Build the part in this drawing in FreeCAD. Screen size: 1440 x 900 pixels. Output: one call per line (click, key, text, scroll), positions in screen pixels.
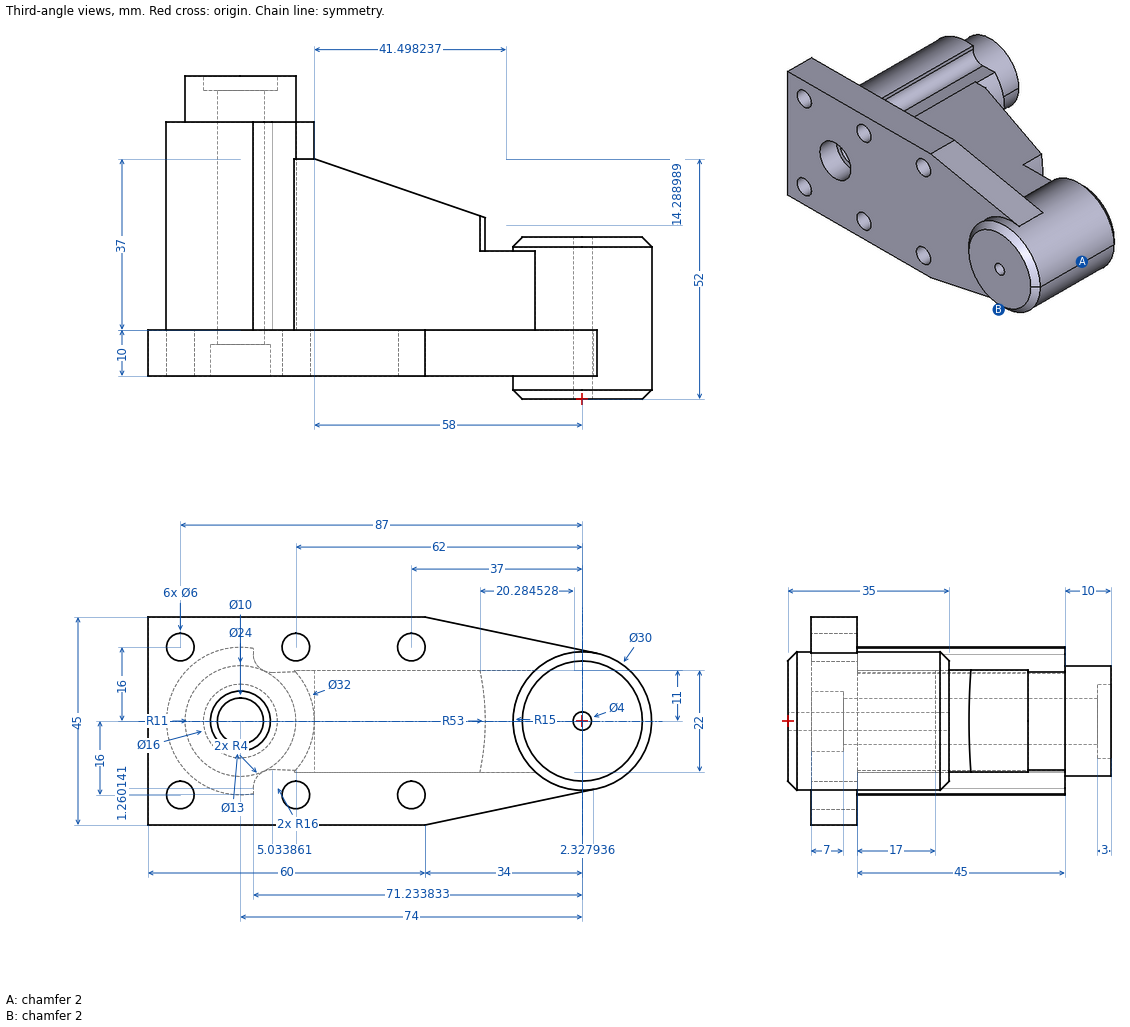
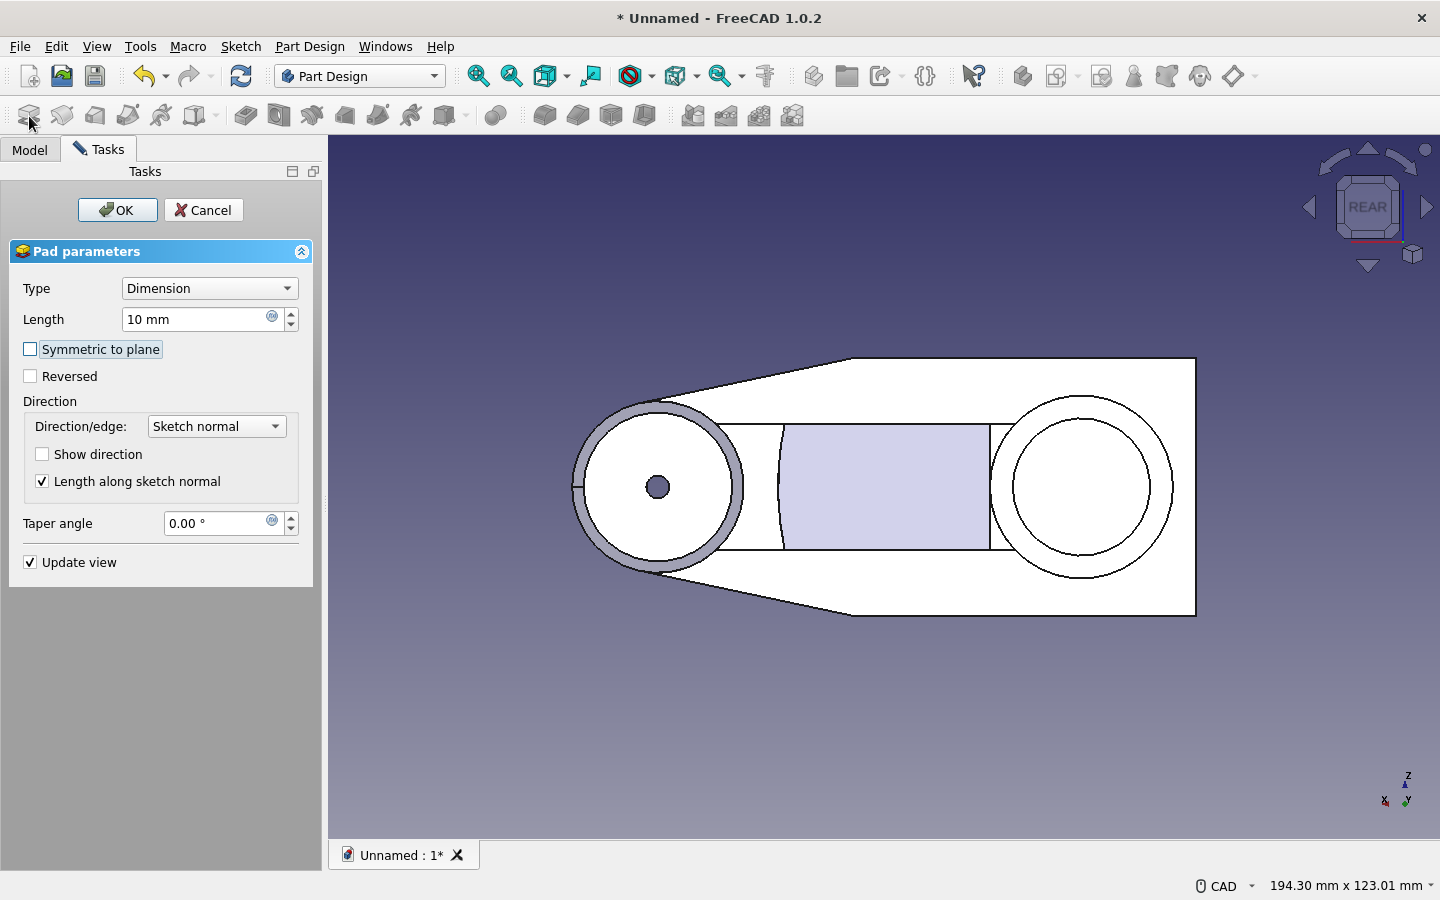
click(118, 210)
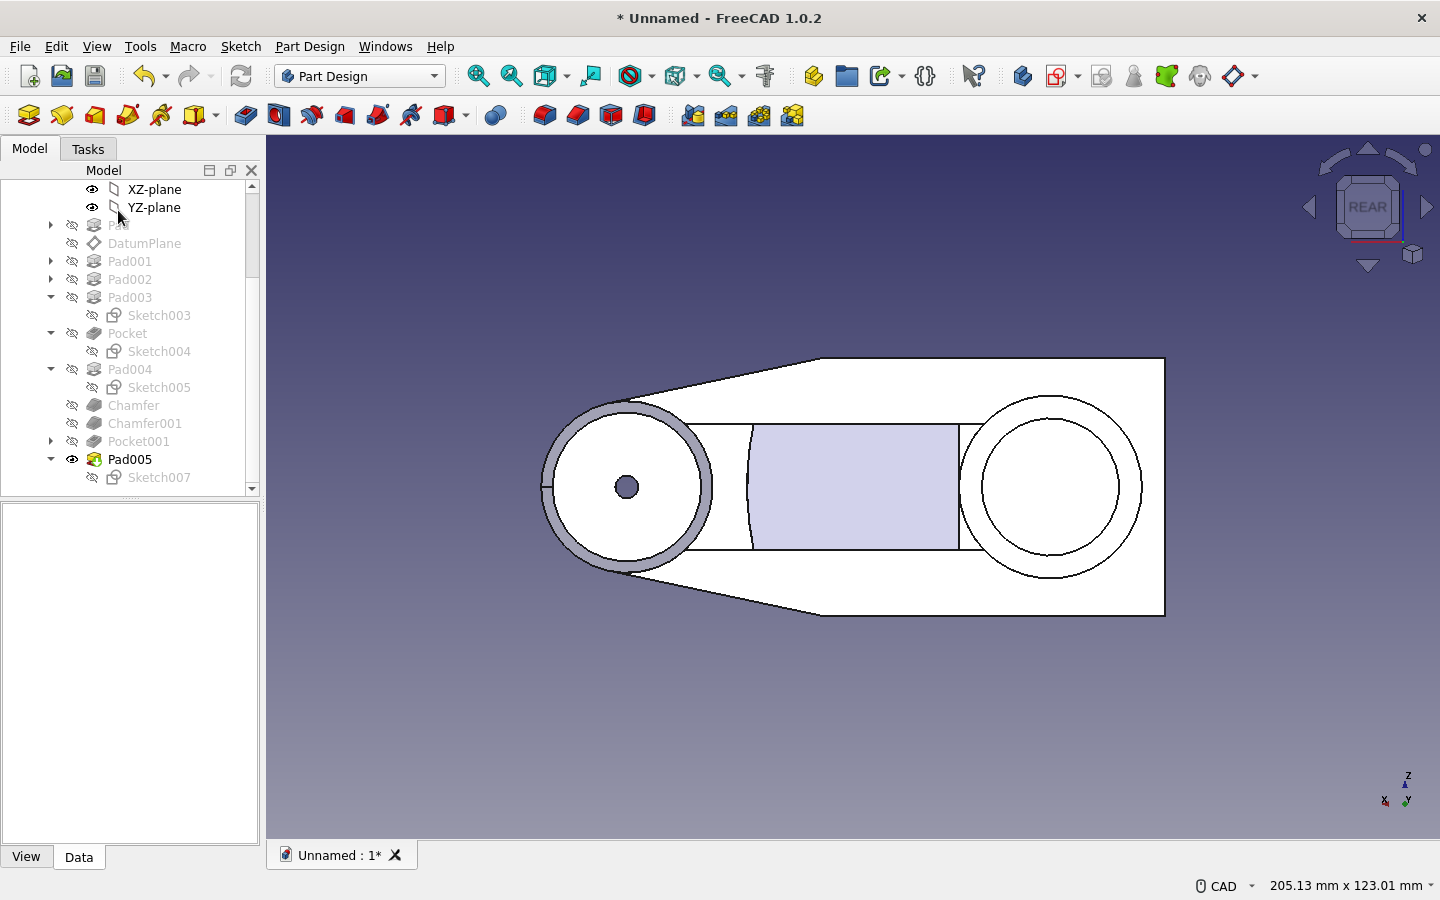
click(1050, 486)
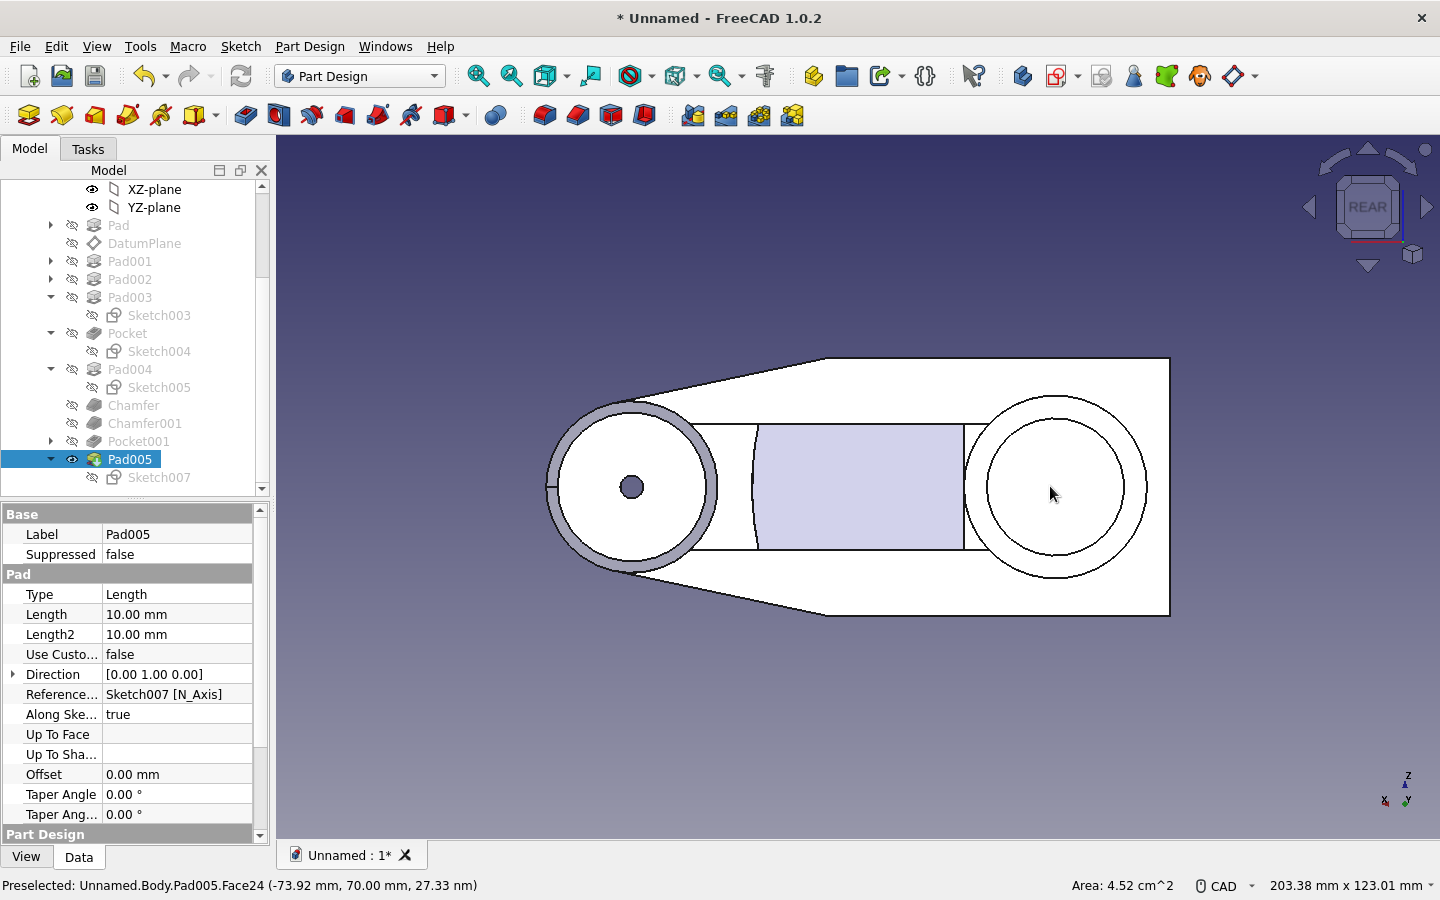
click(1056, 76)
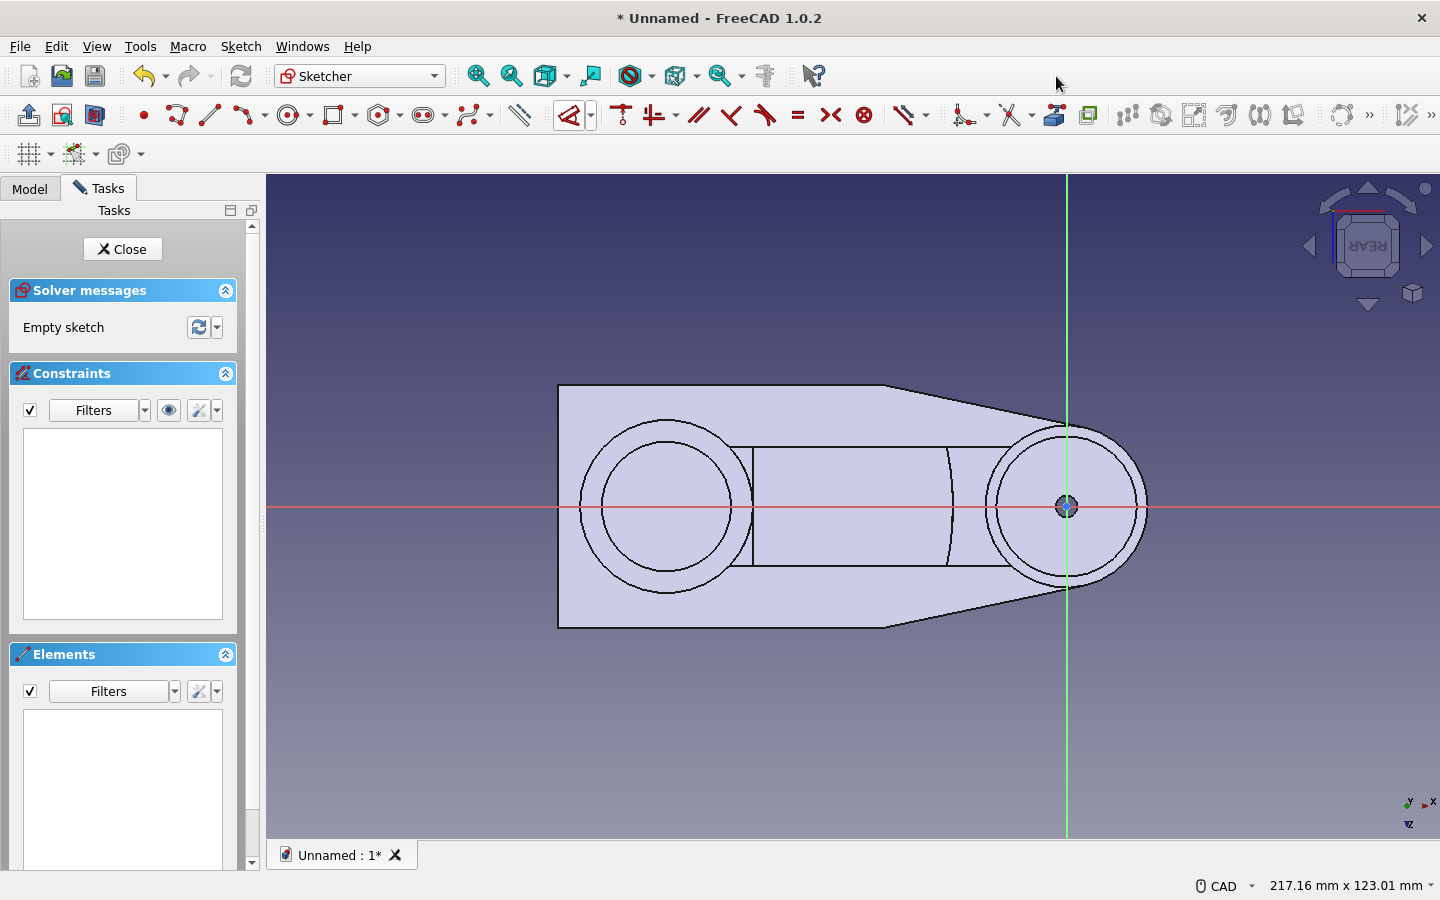
scroll(637, 506, up, 8)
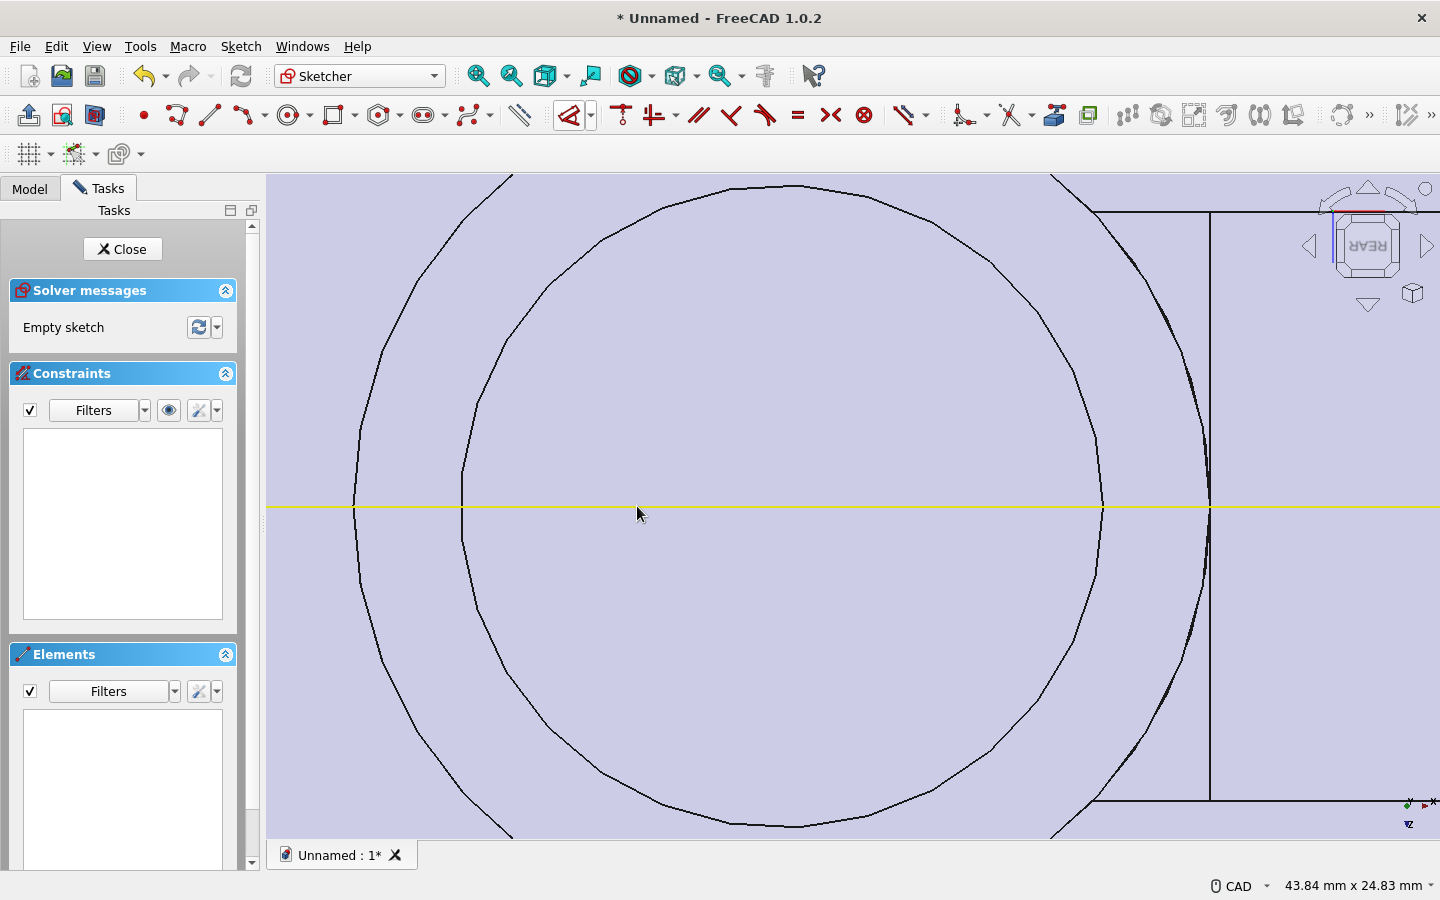
click(288, 116)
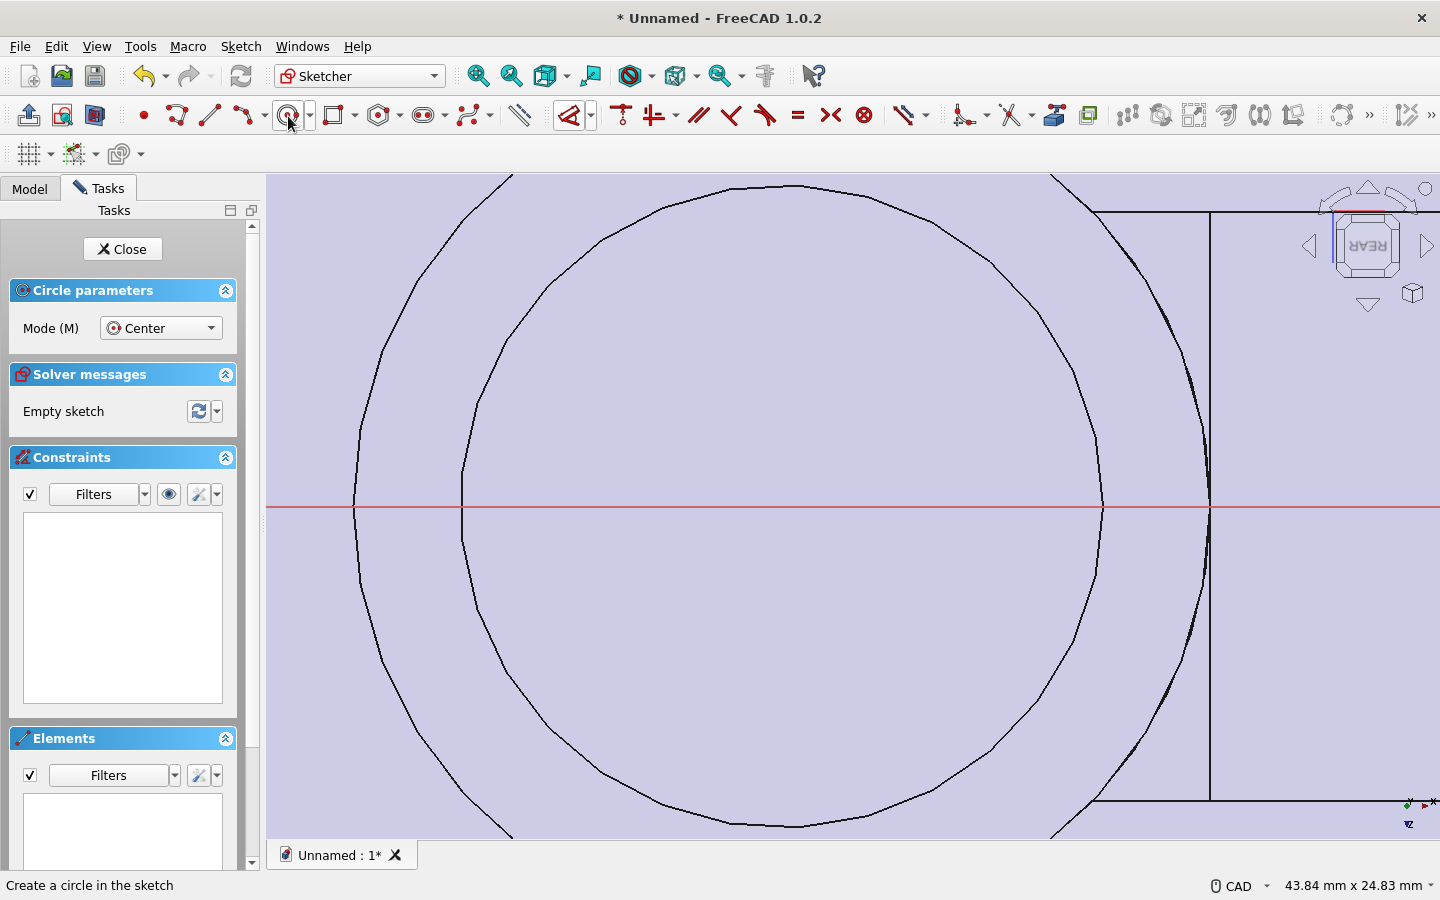
click(782, 506)
click(933, 355)
key(Escape)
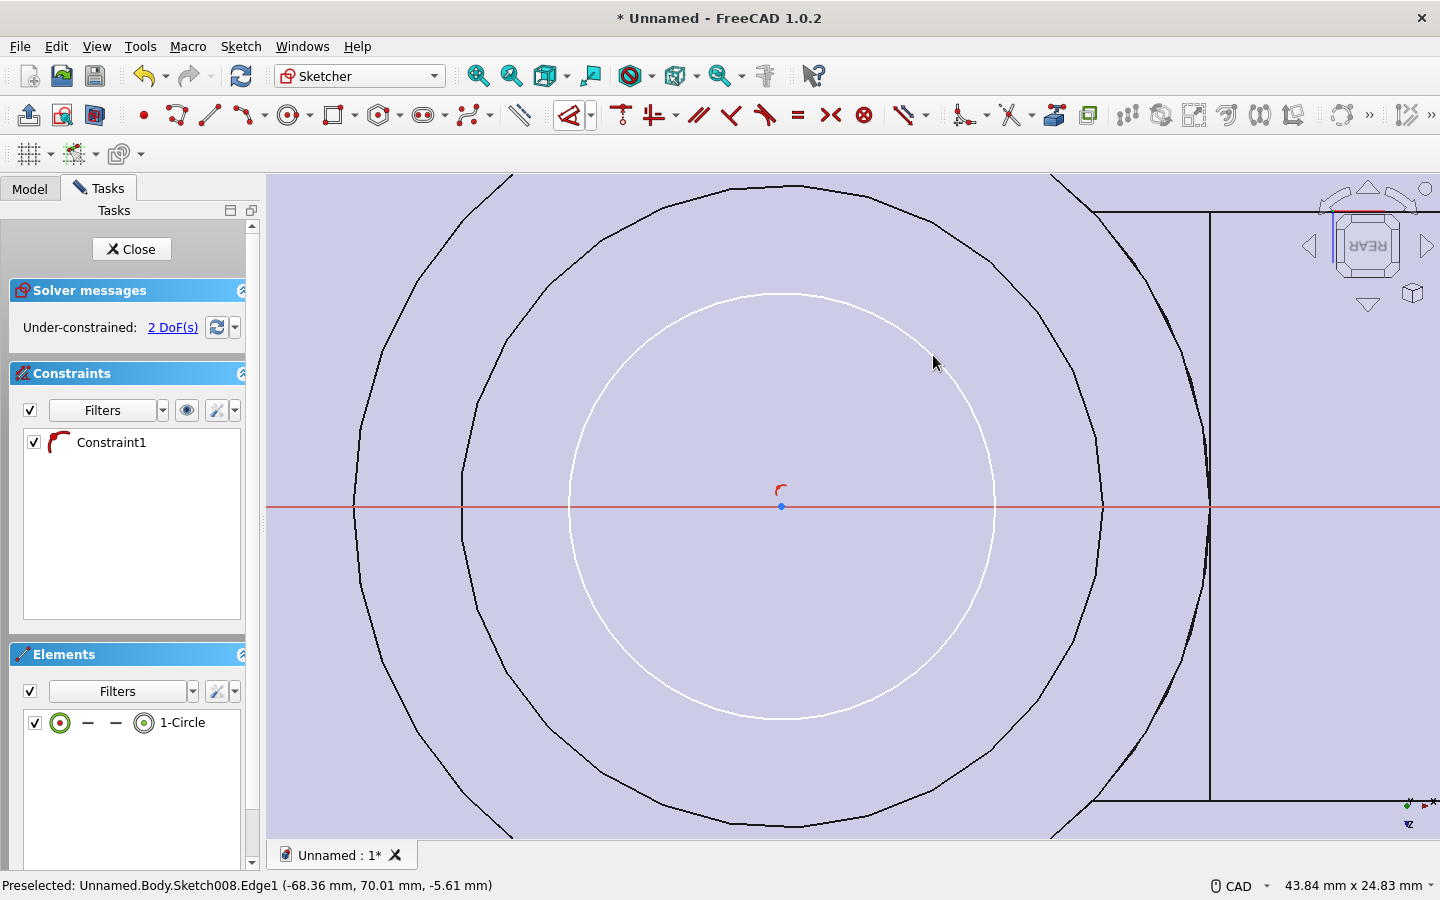
click(932, 355)